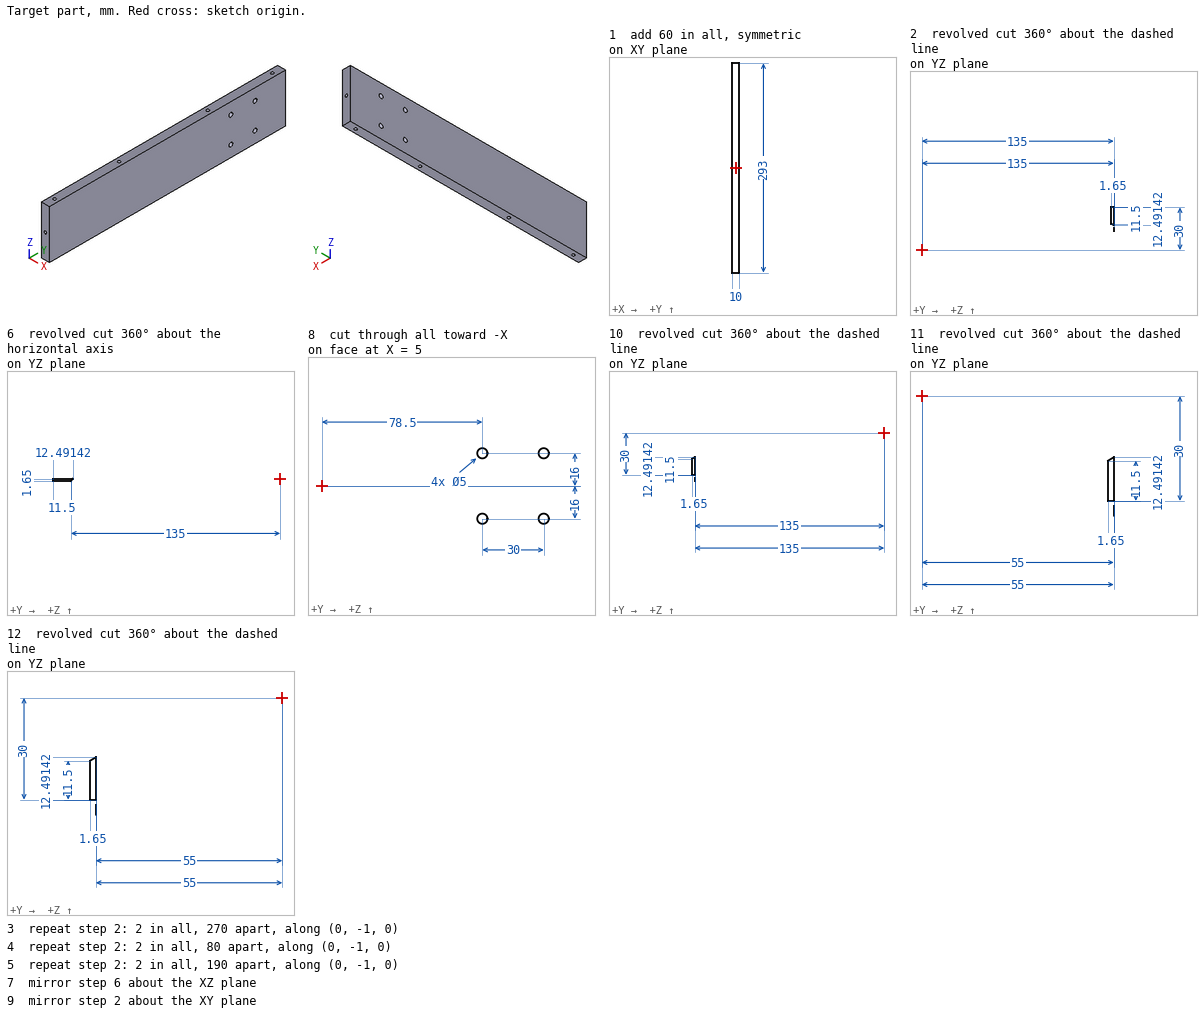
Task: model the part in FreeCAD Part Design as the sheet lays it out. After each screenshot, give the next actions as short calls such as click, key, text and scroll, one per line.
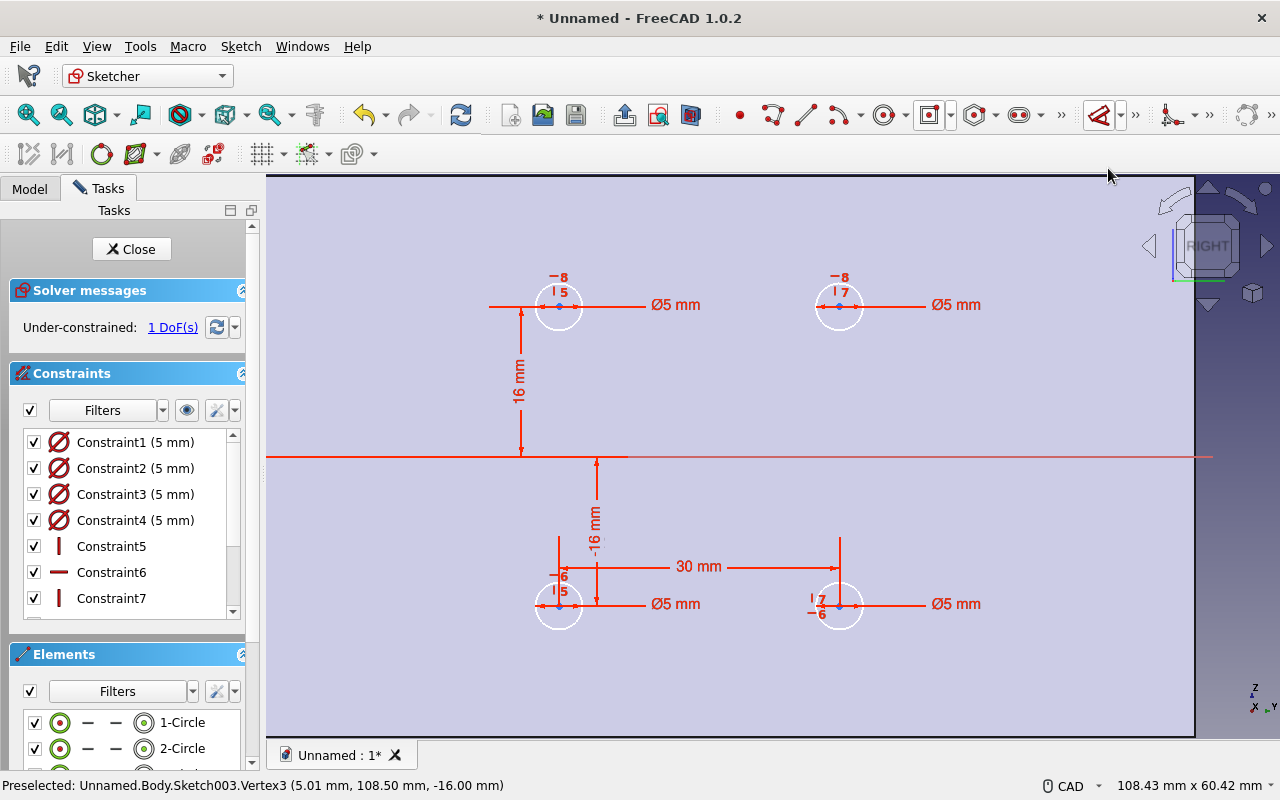
click(559, 307)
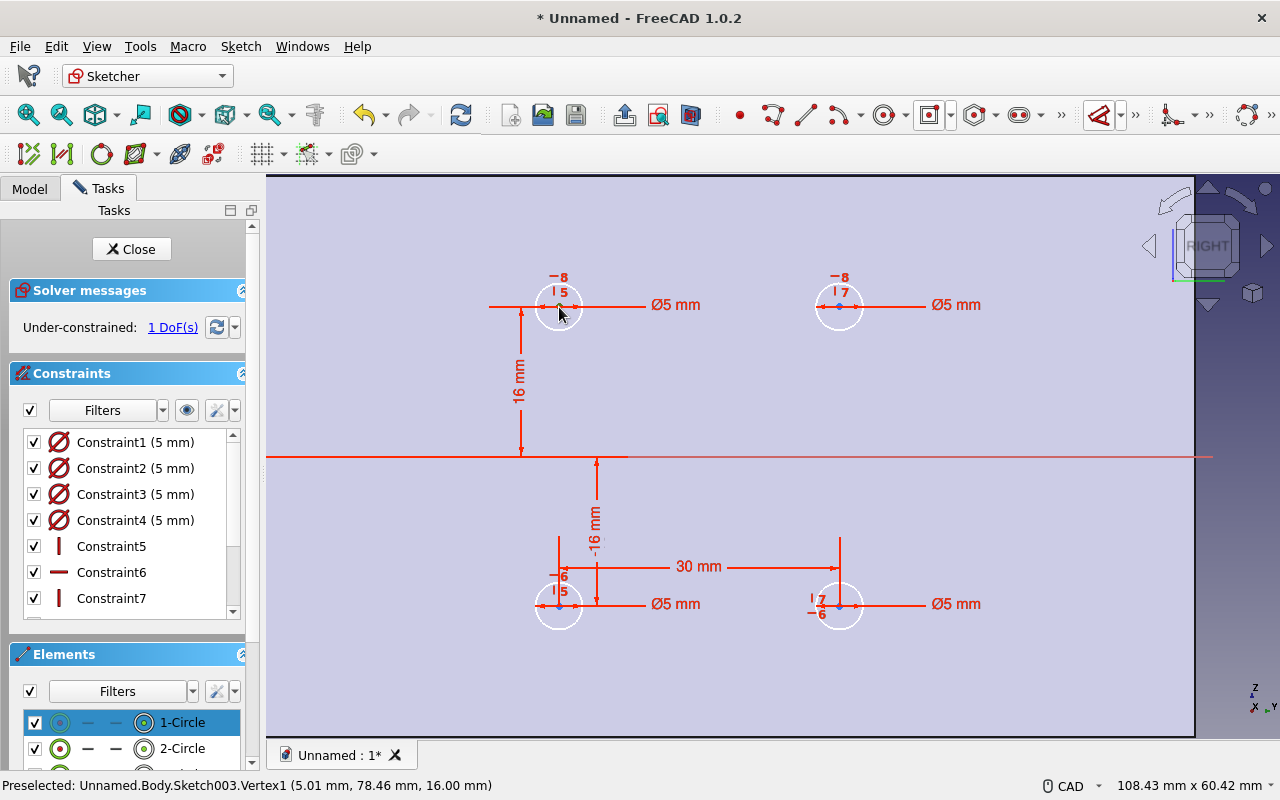
click(1120, 116)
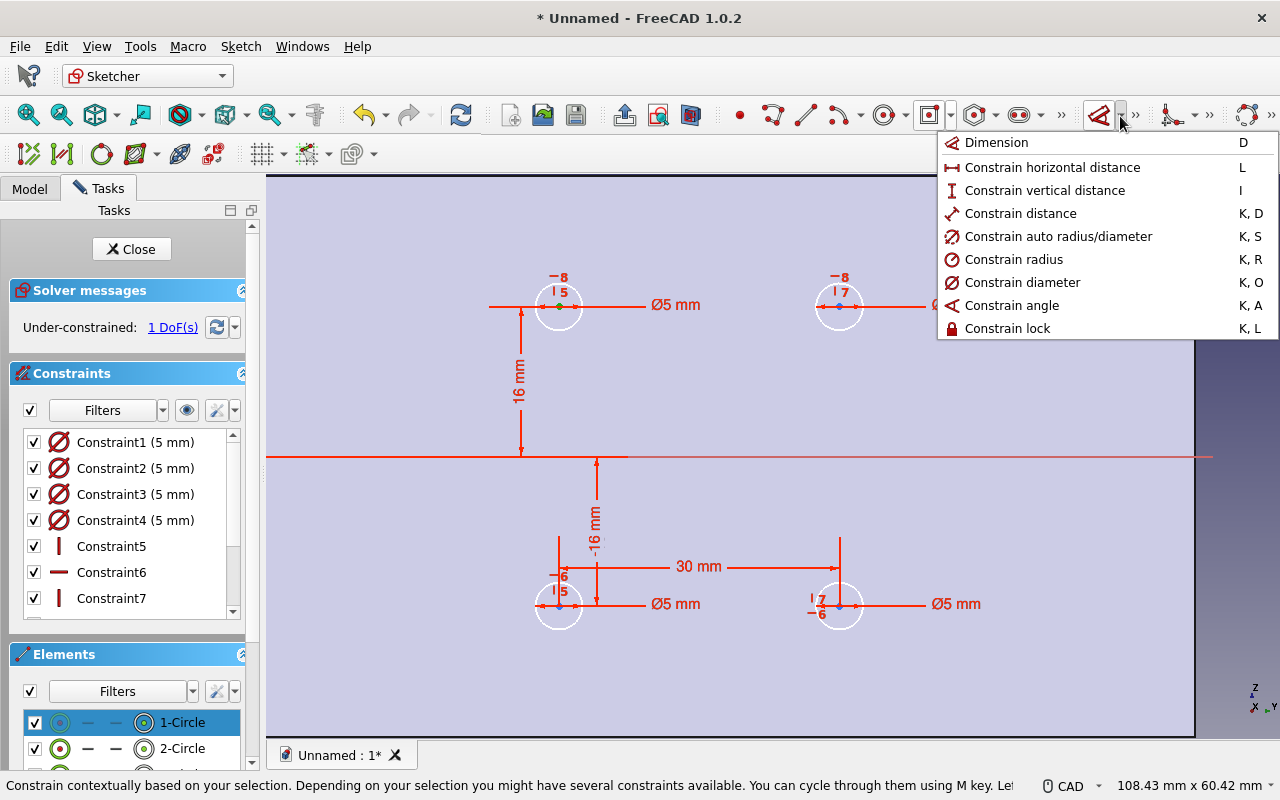
click(1108, 168)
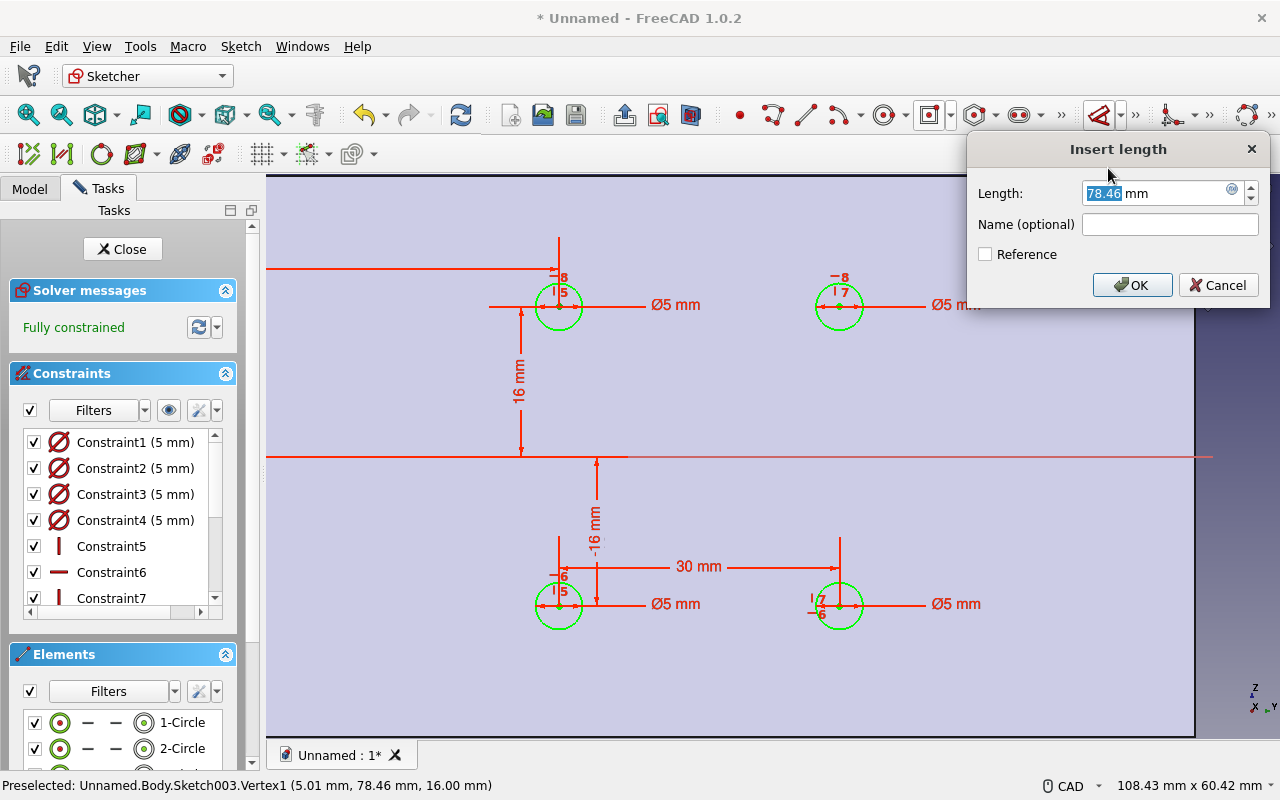
text(78.5)
key(Return)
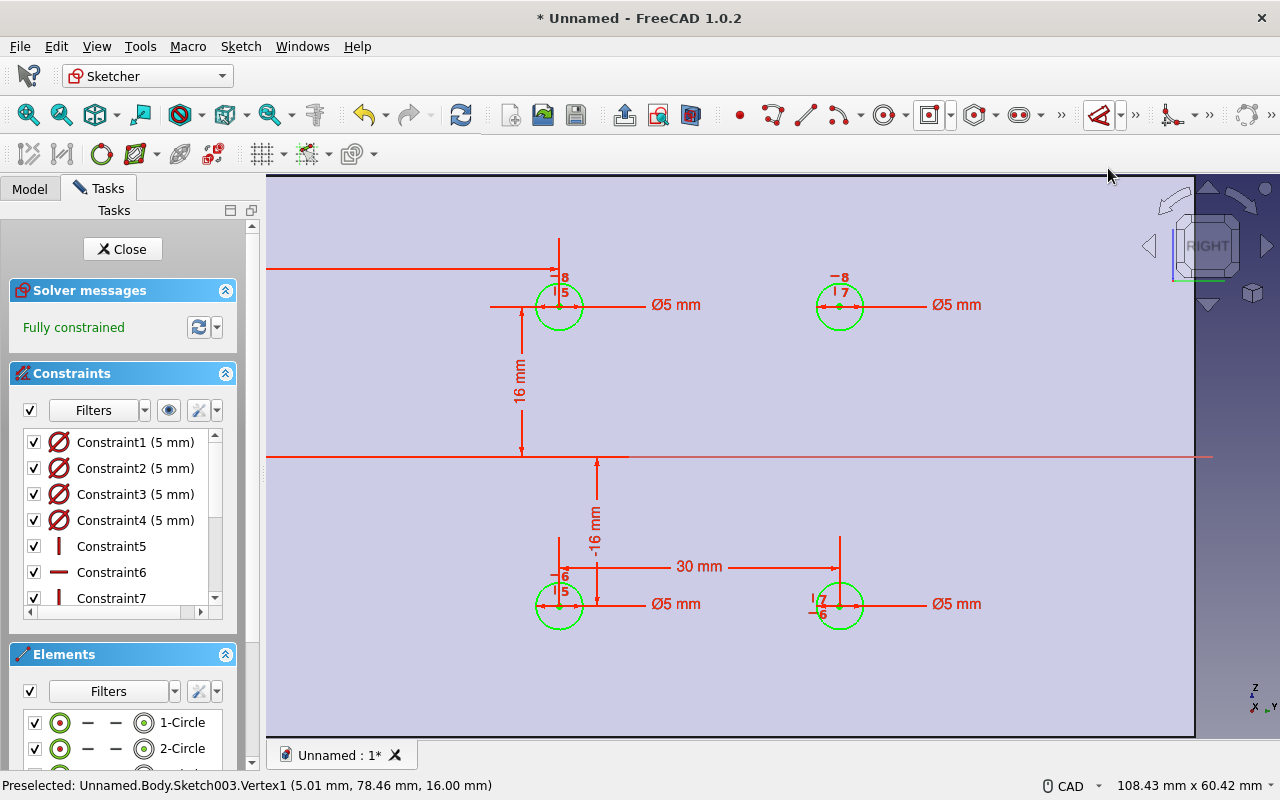
click(123, 249)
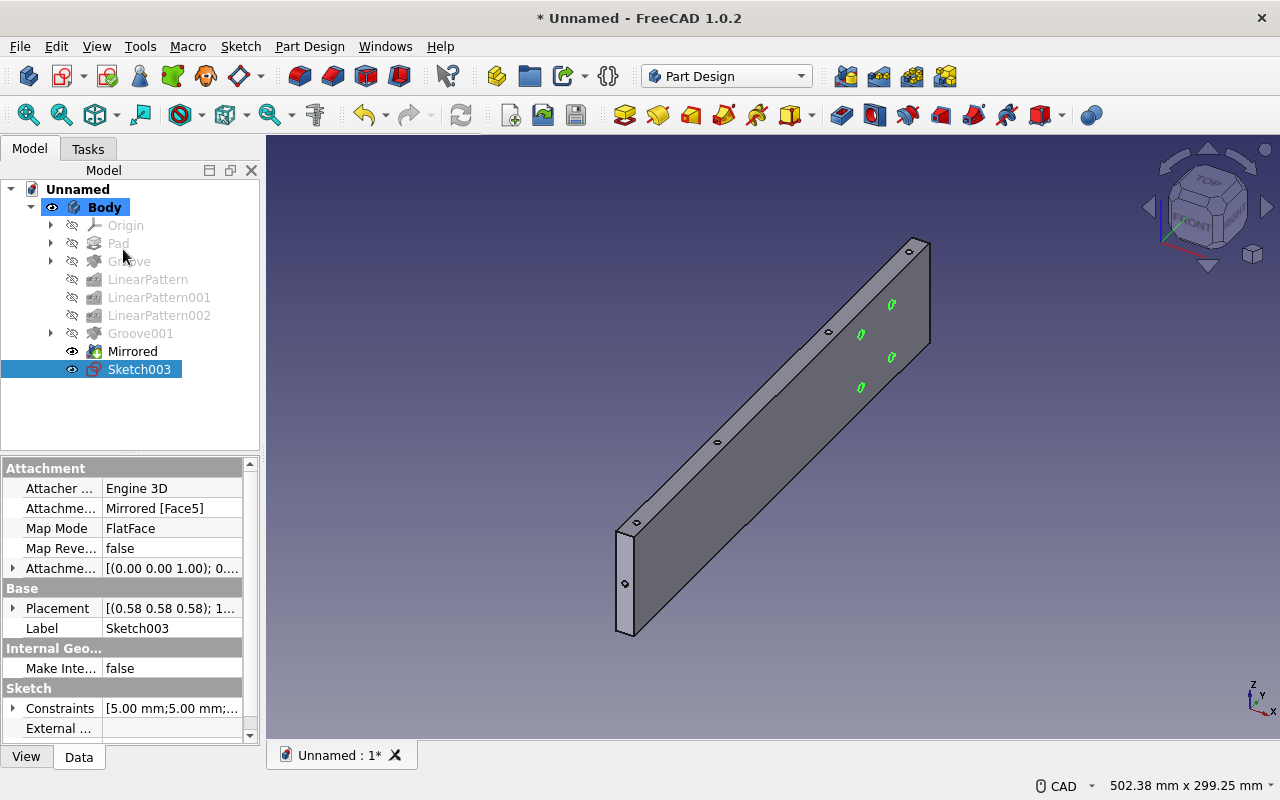
click(842, 116)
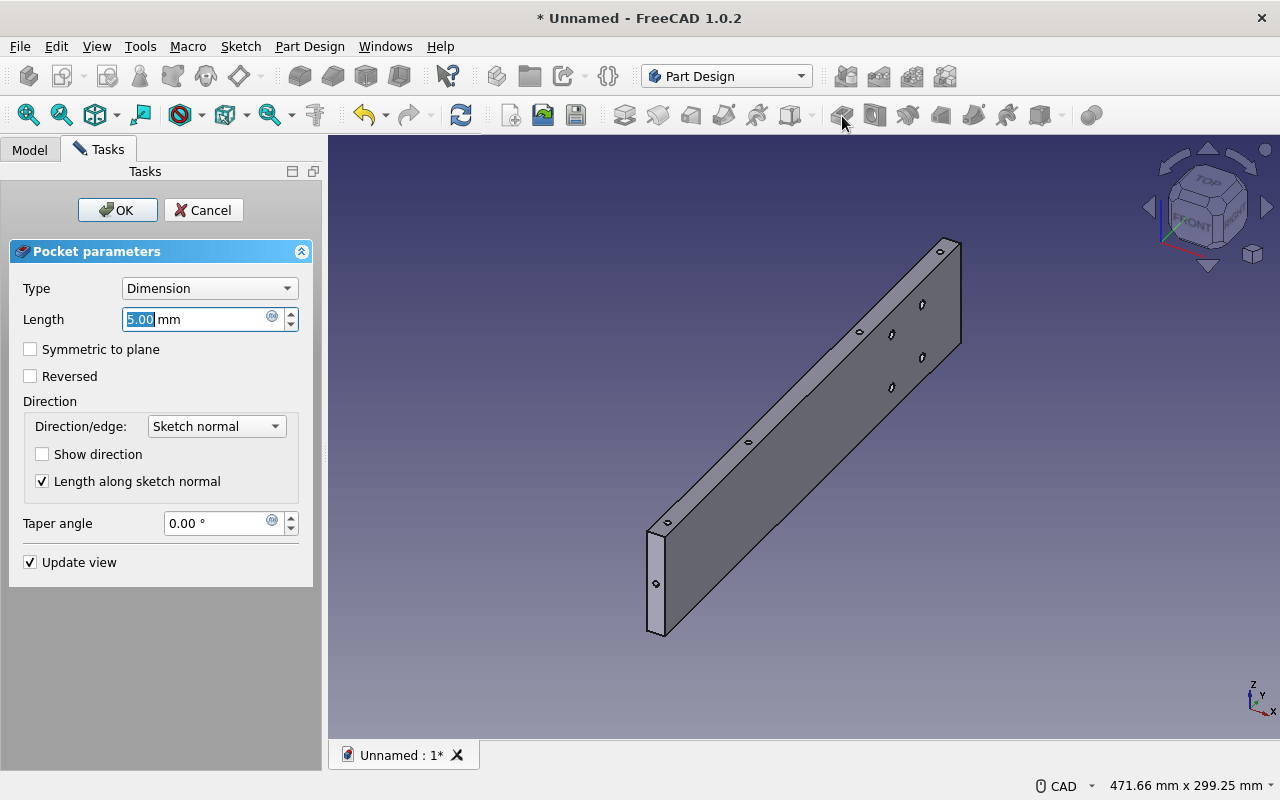
click(210, 288)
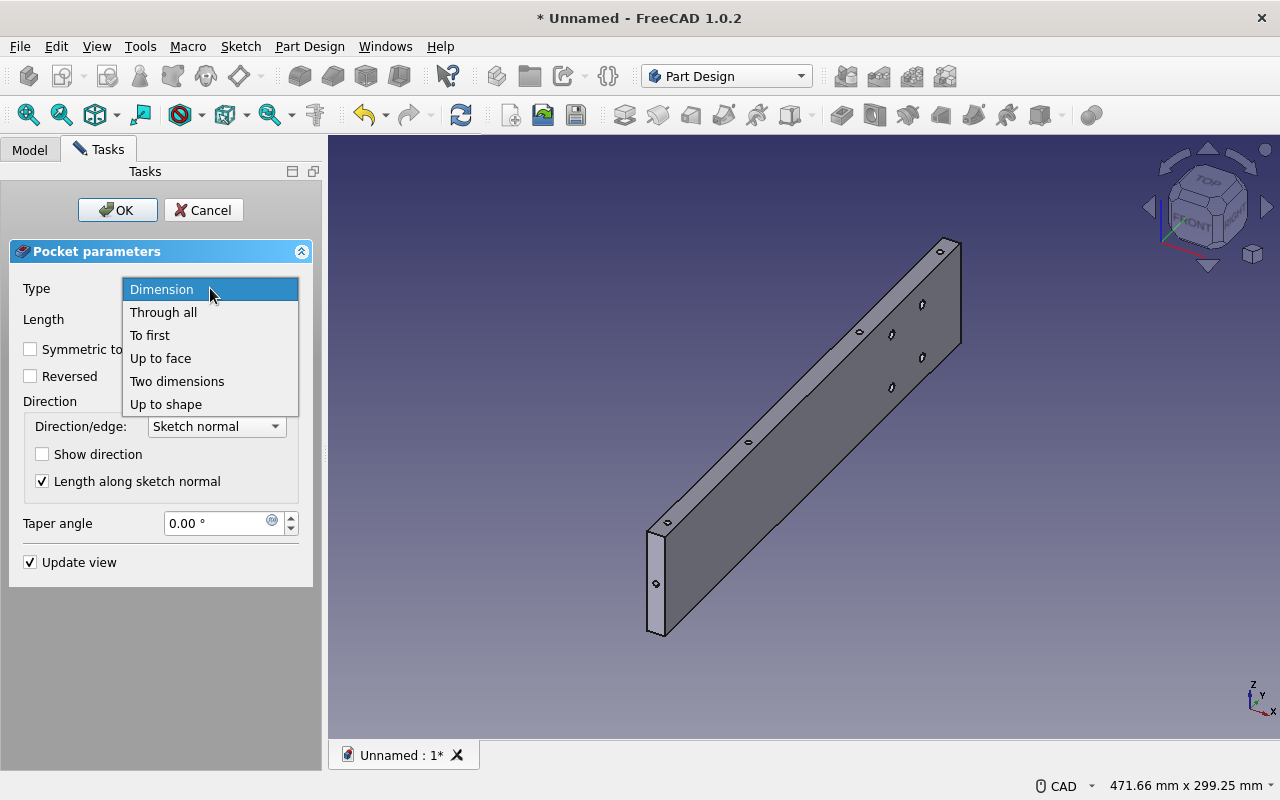
click(208, 312)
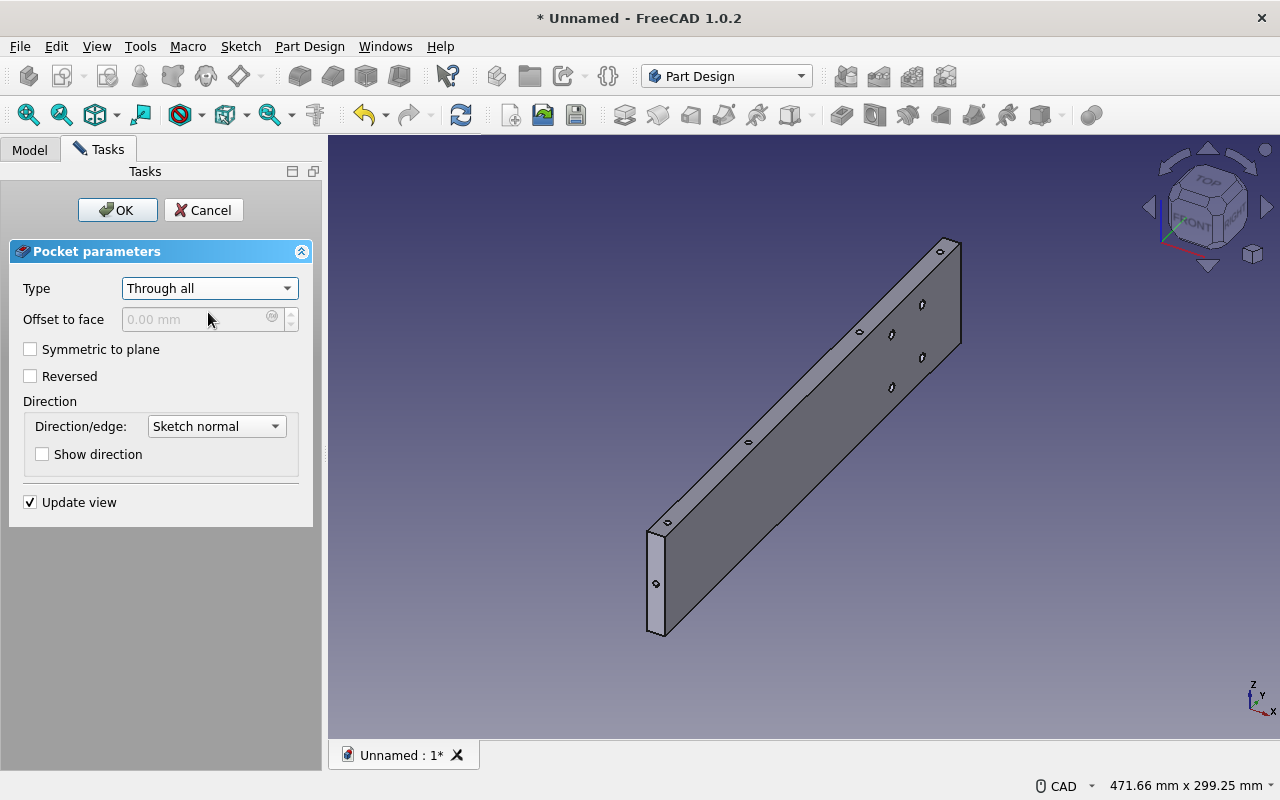
click(118, 210)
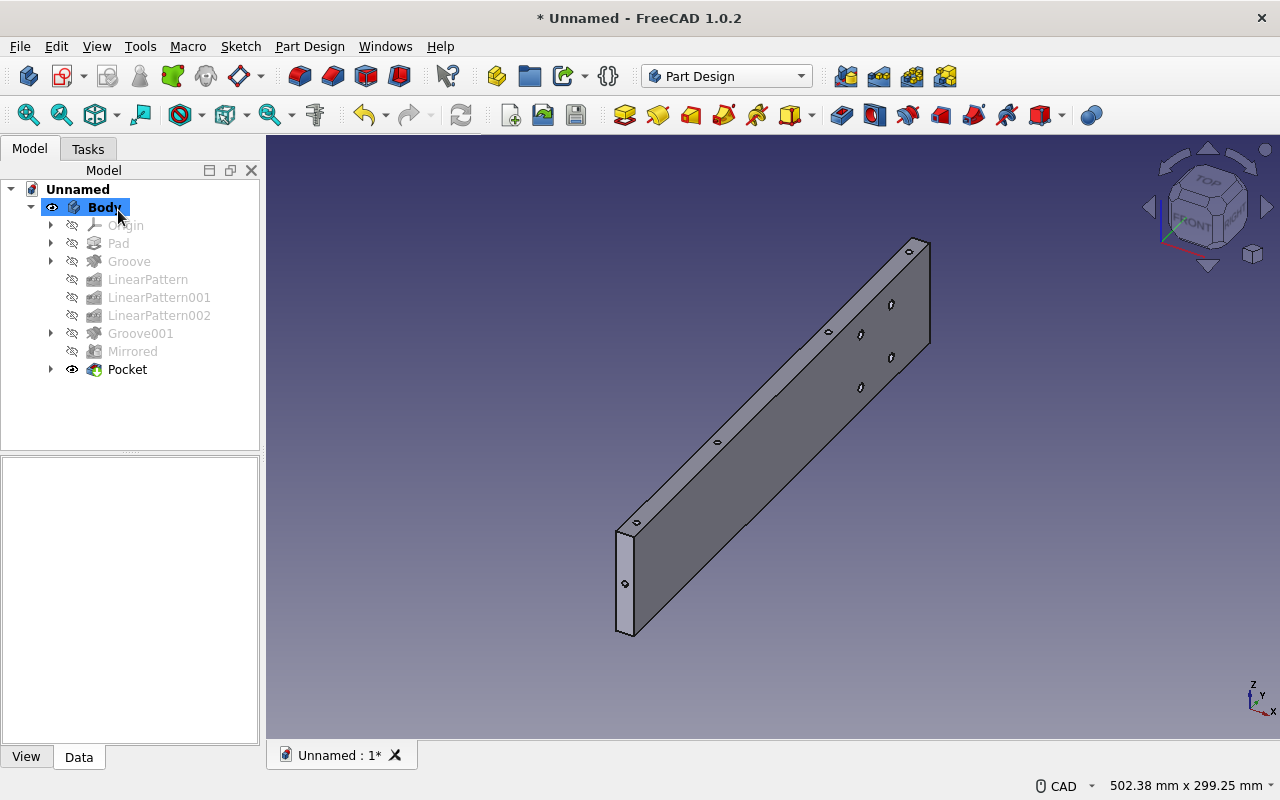
click(117, 261)